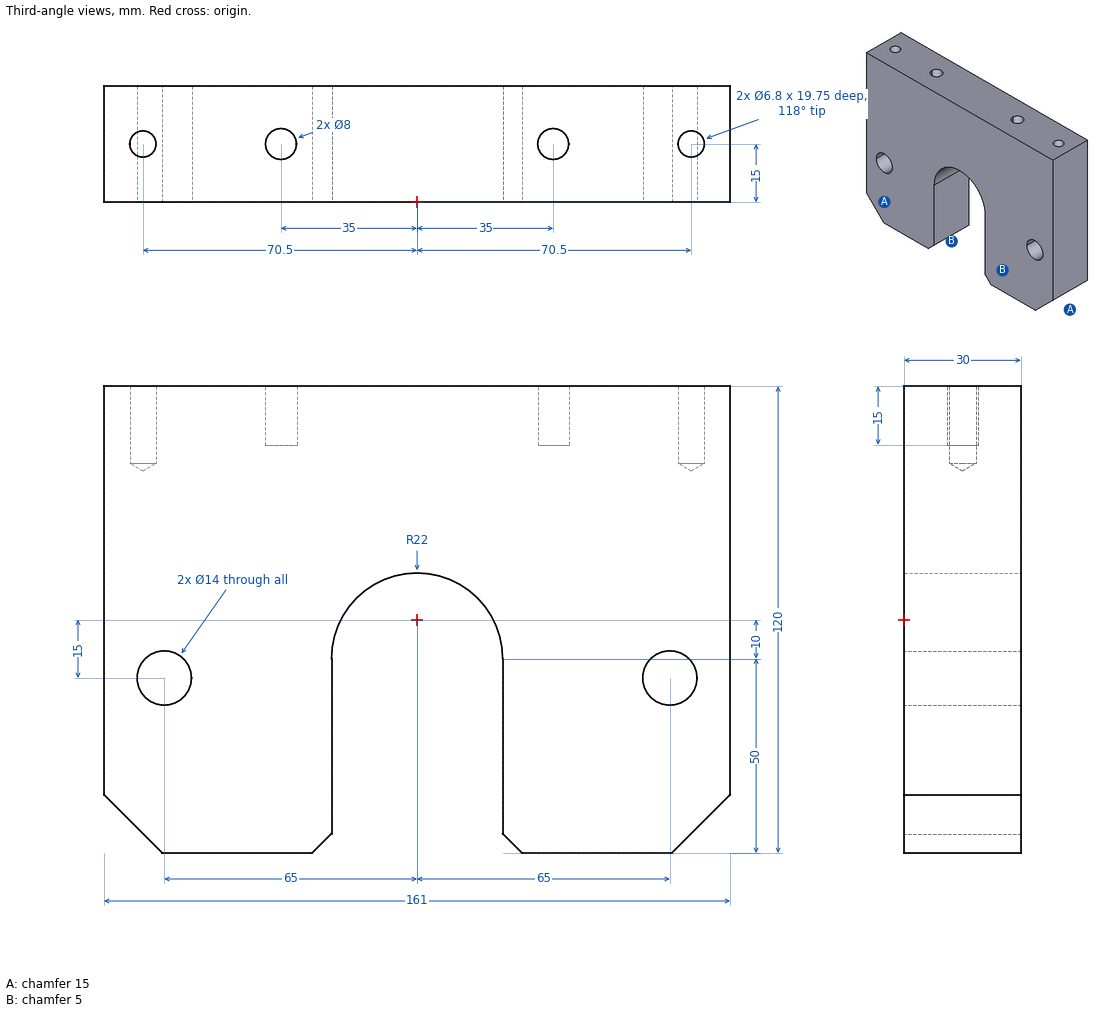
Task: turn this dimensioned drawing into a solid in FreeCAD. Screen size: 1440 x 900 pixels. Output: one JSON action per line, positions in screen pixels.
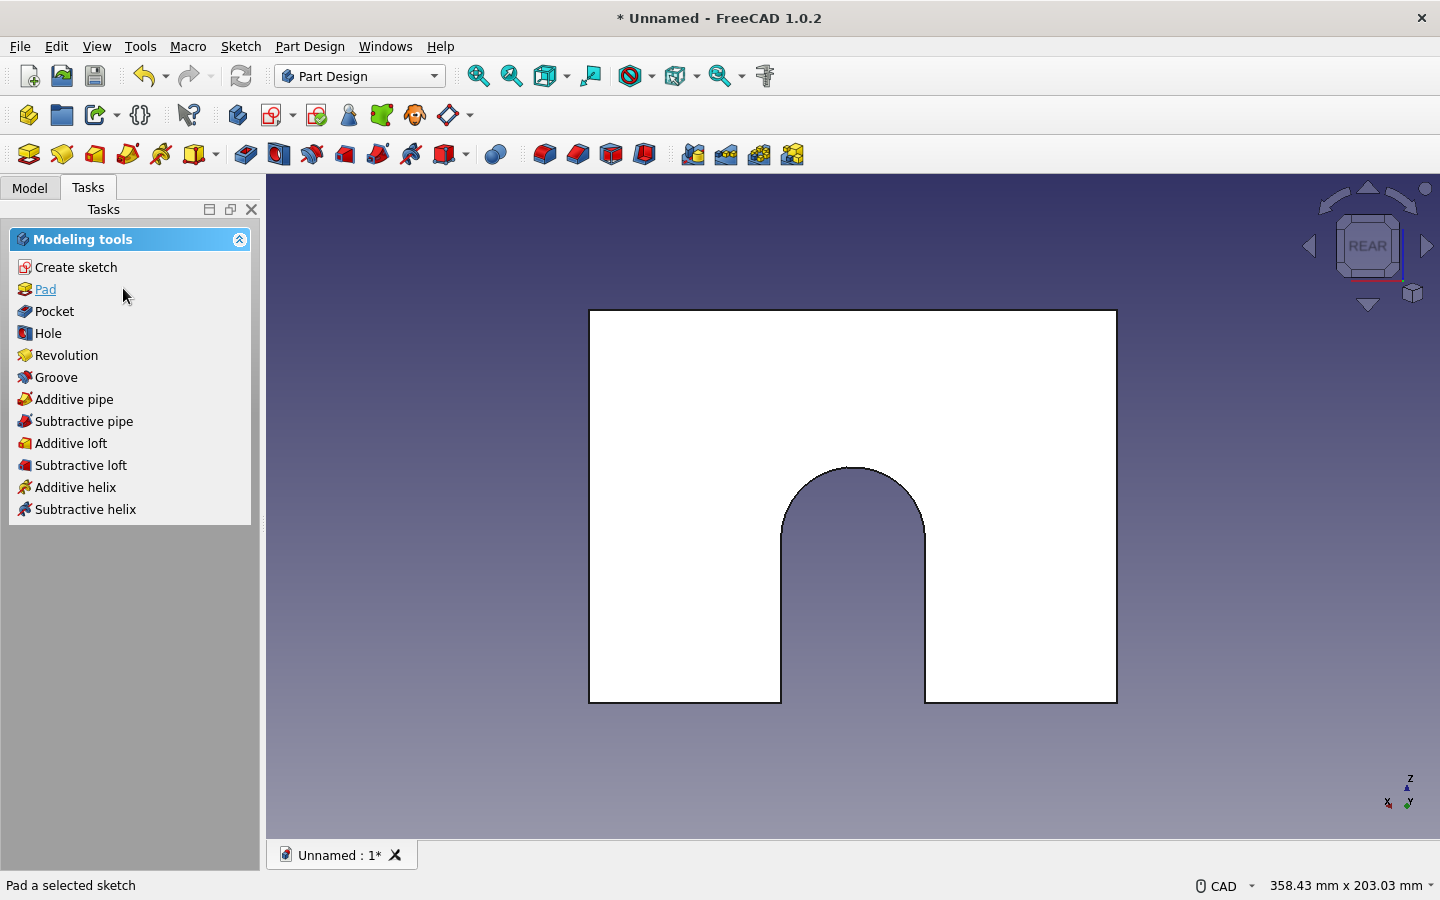
{"action": "left_click", "coordinate": [279, 154]}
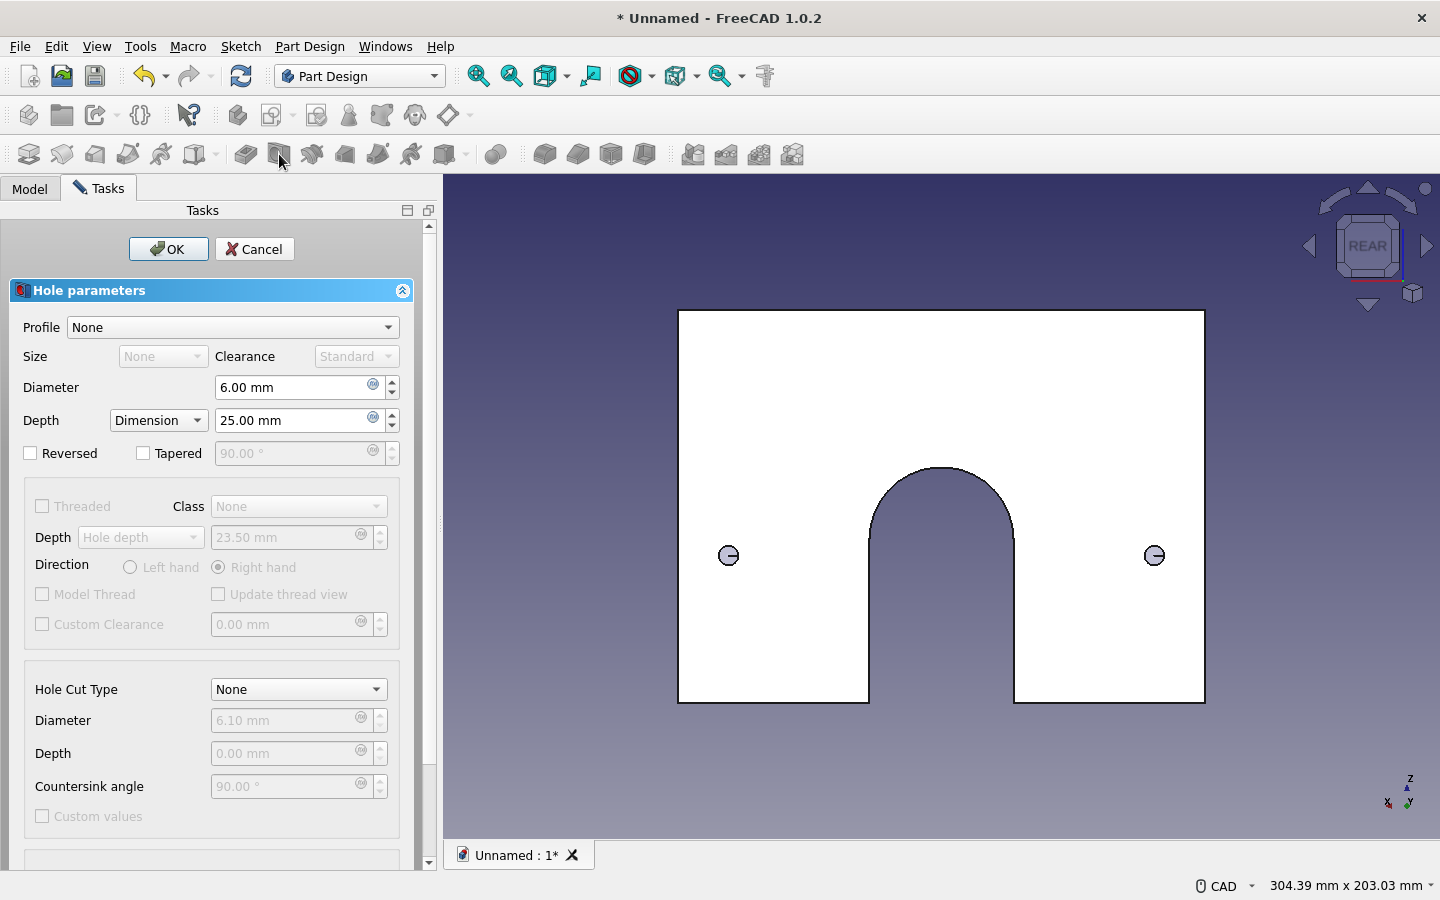
{"action": "triple_click", "coordinate": [300, 388]}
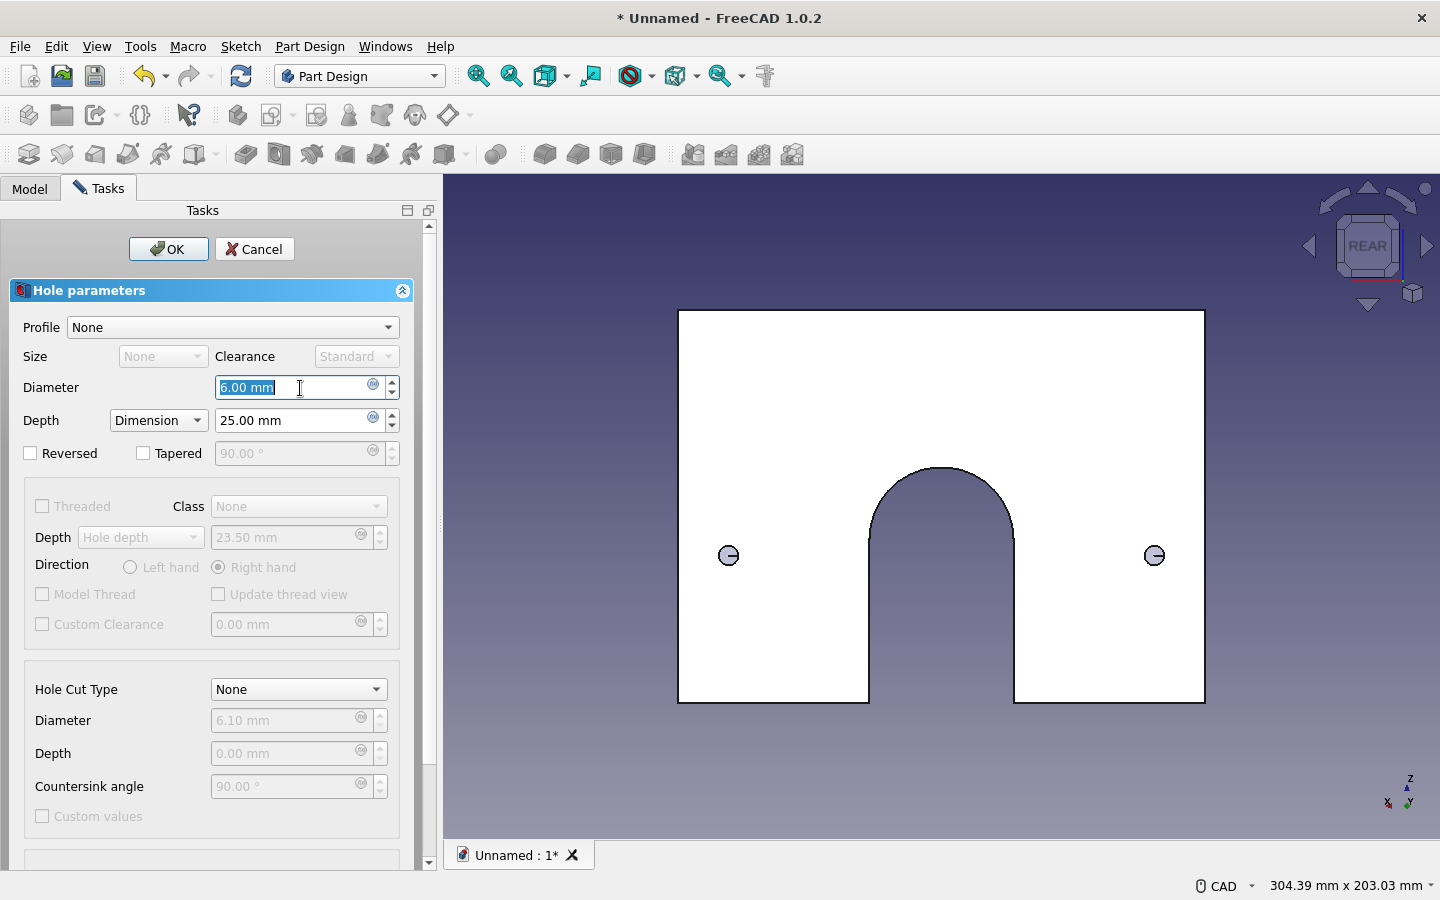
{"action": "type", "text": "14"}
{"action": "key", "text": "Tab"}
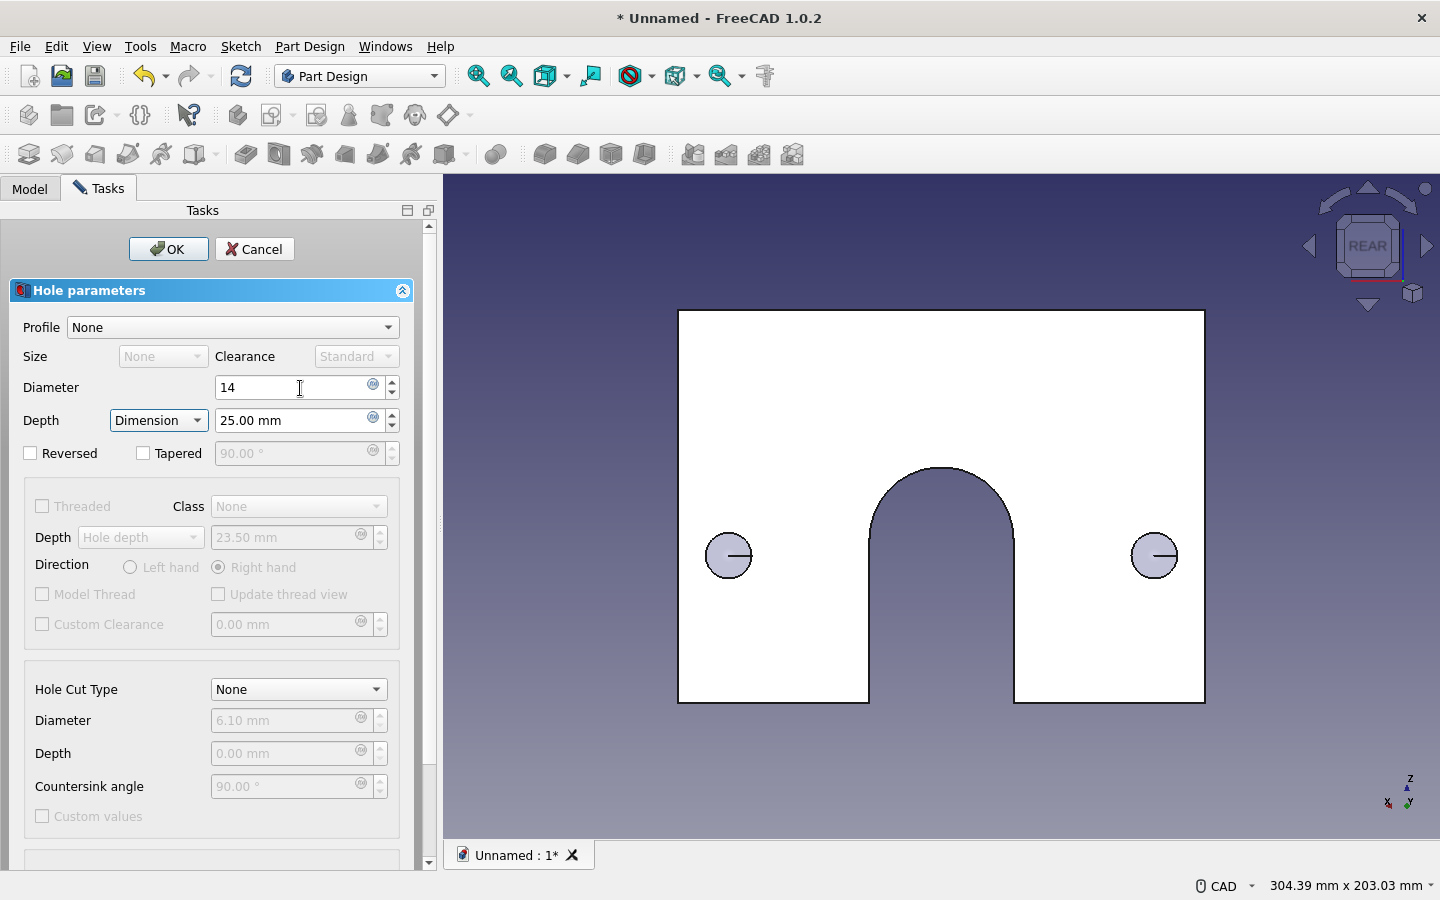
{"action": "left_click", "coordinate": [160, 420]}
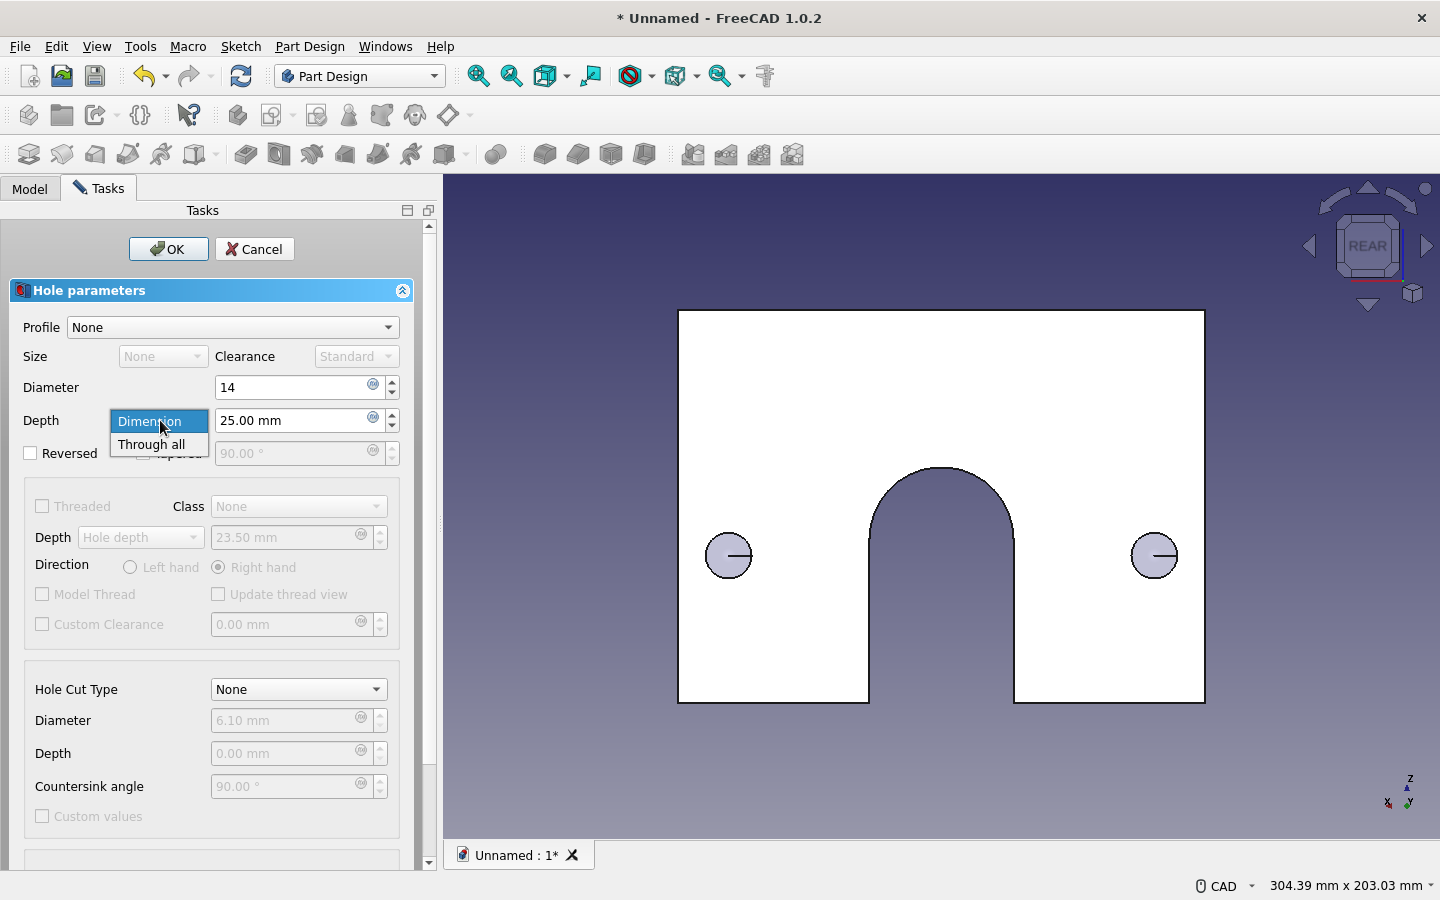
{"action": "left_click", "coordinate": [158, 444]}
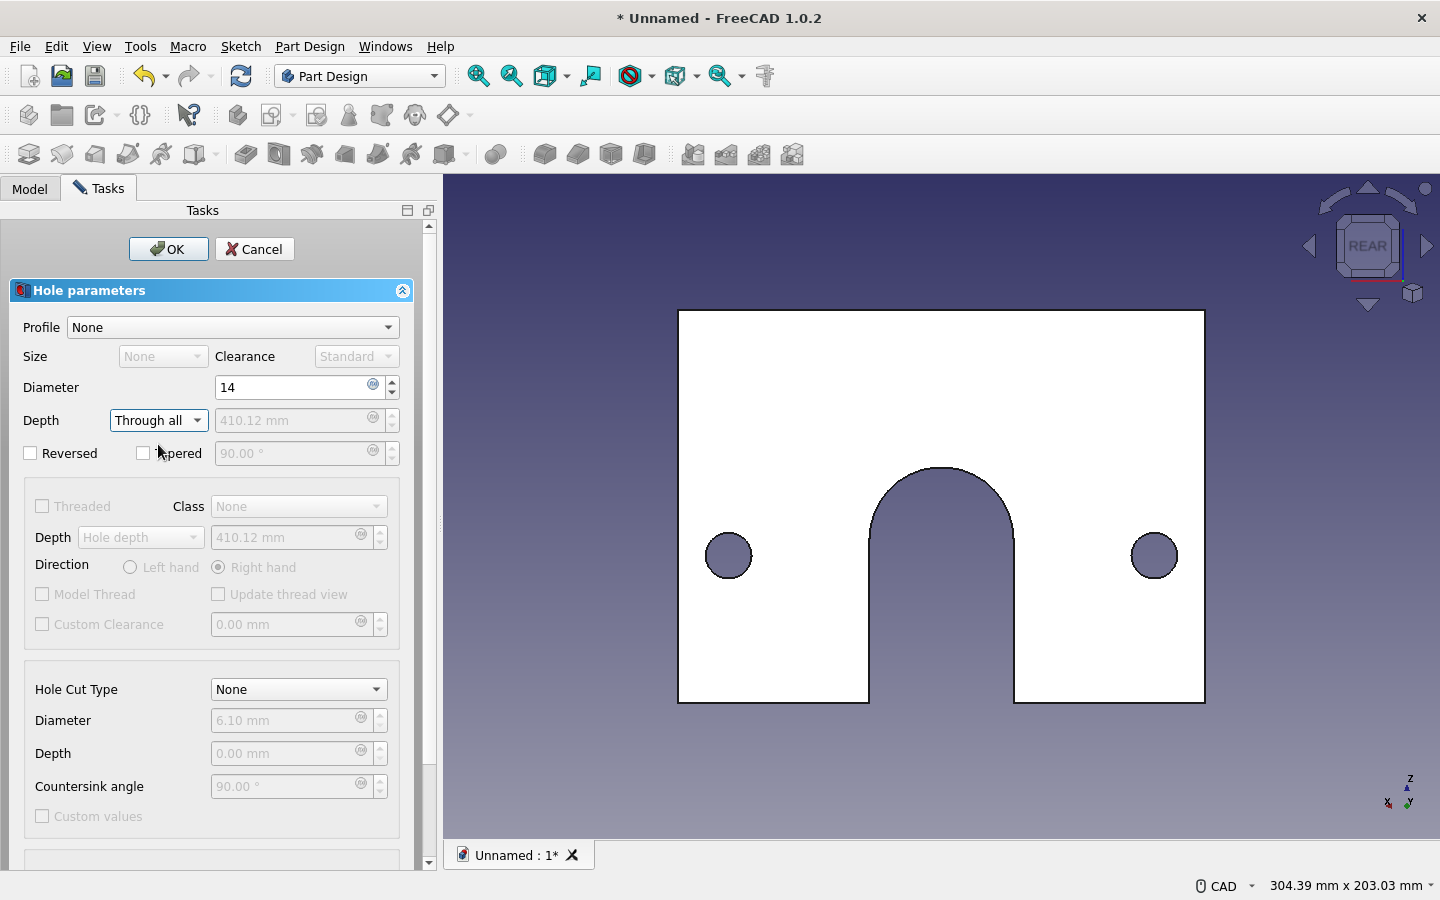
{"action": "left_click", "coordinate": [169, 249]}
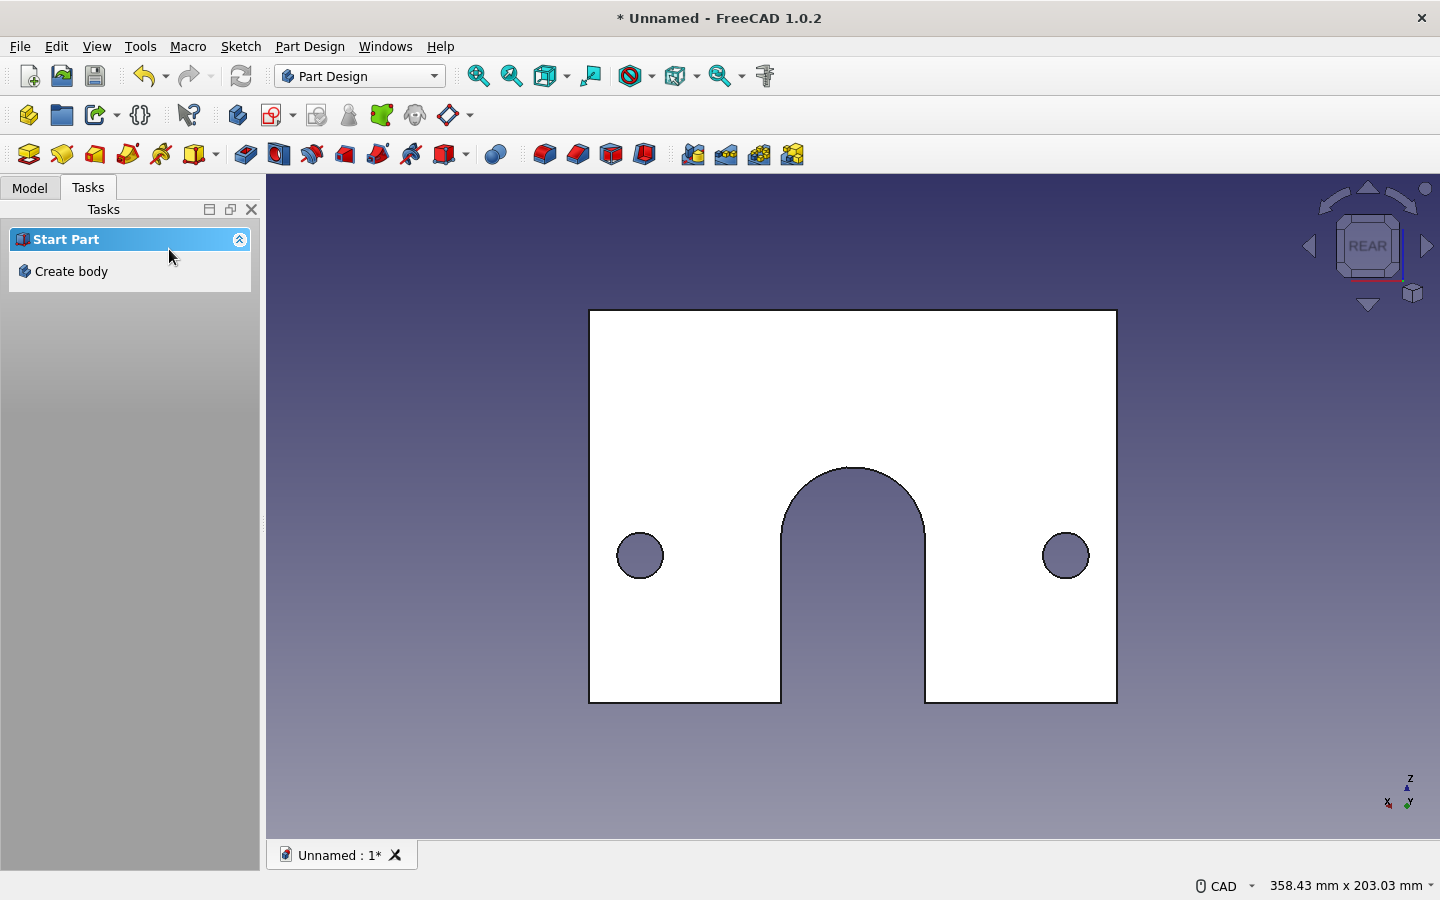
{"action": "key", "text": "0"}